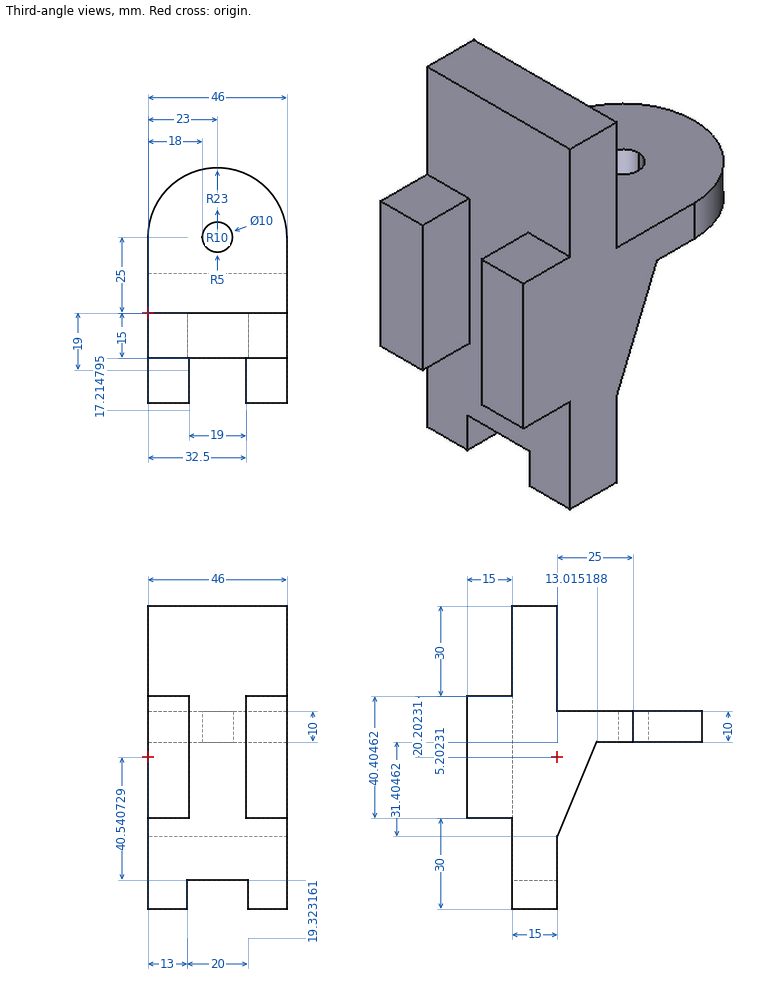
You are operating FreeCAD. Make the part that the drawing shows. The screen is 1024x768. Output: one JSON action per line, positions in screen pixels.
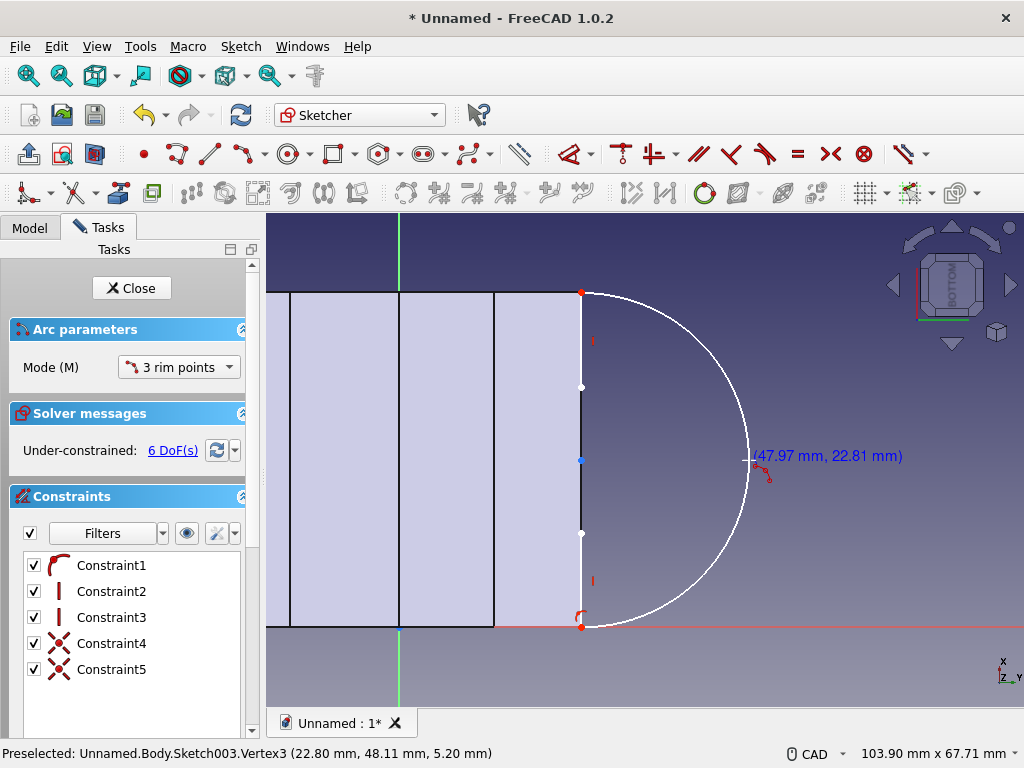
{"action": "left_click", "coordinate": [581, 388]}
{"action": "left_click", "coordinate": [581, 534]}
{"action": "left_click", "coordinate": [654, 460]}
{"action": "key", "text": "Escape"}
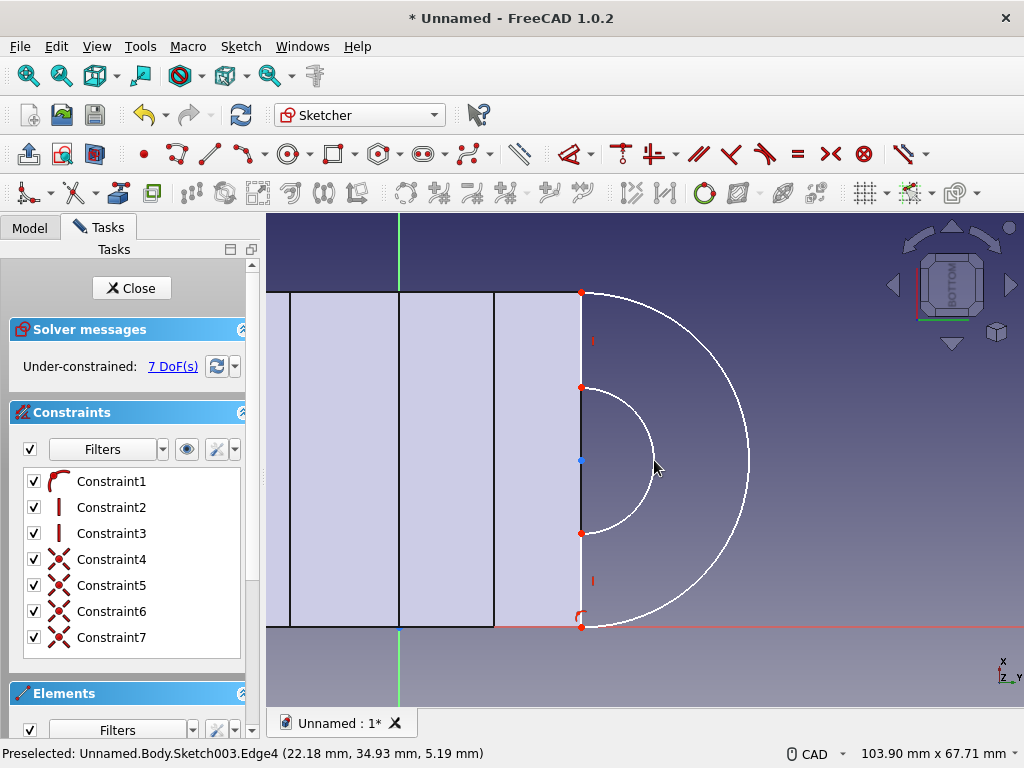
{"action": "left_click", "coordinate": [717, 559]}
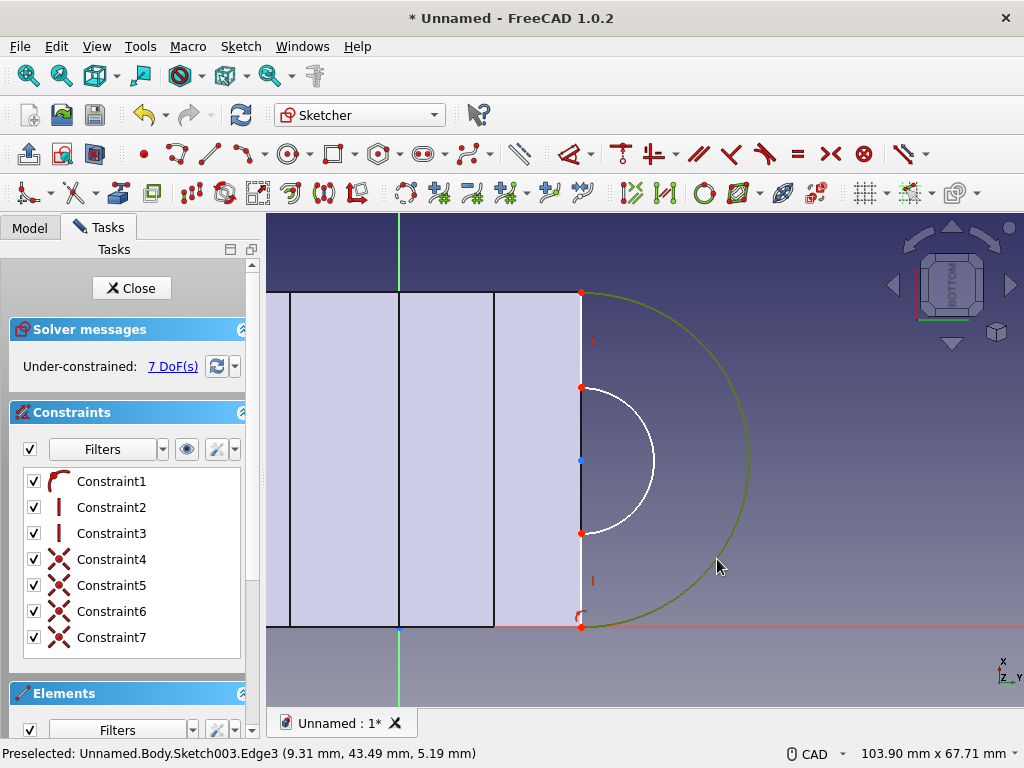
{"action": "left_click", "coordinate": [640, 504]}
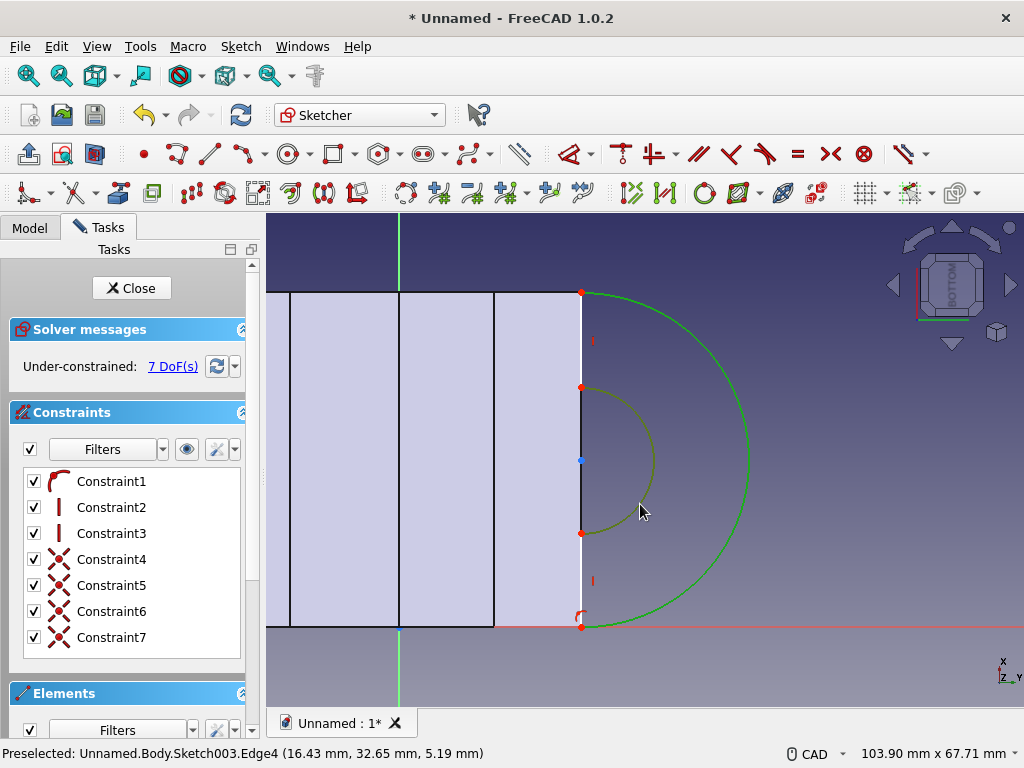
{"action": "key", "text": "c"}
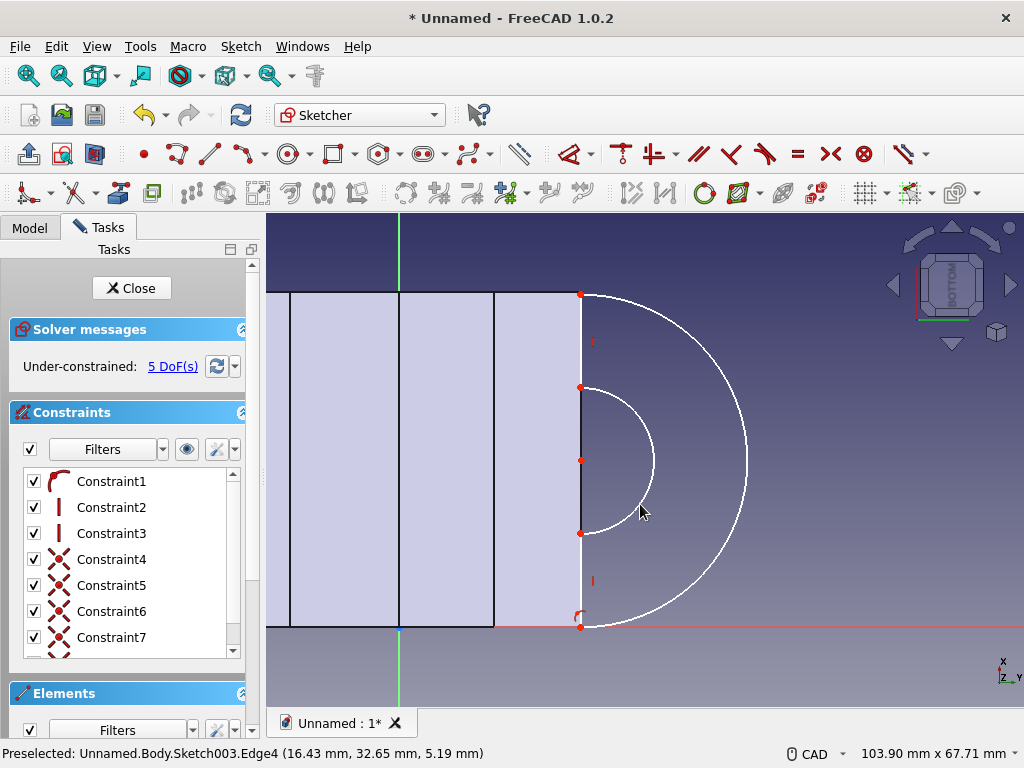
{"action": "left_click", "coordinate": [568, 154]}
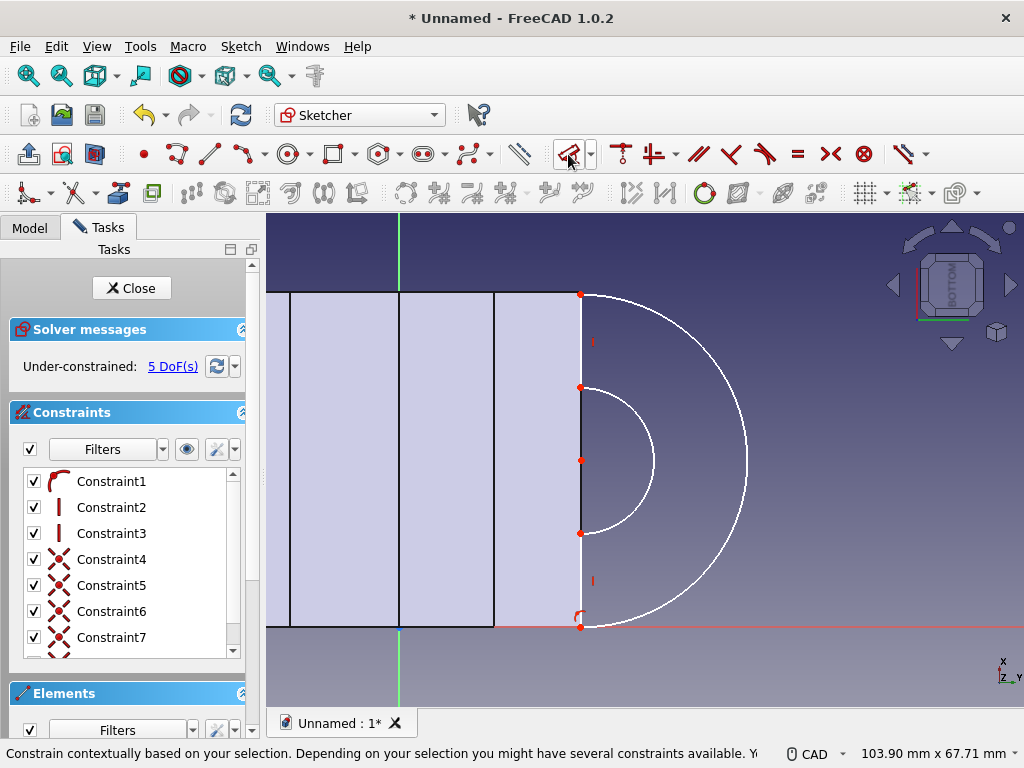
{"action": "left_click", "coordinate": [716, 559]}
{"action": "left_click", "coordinate": [742, 578]}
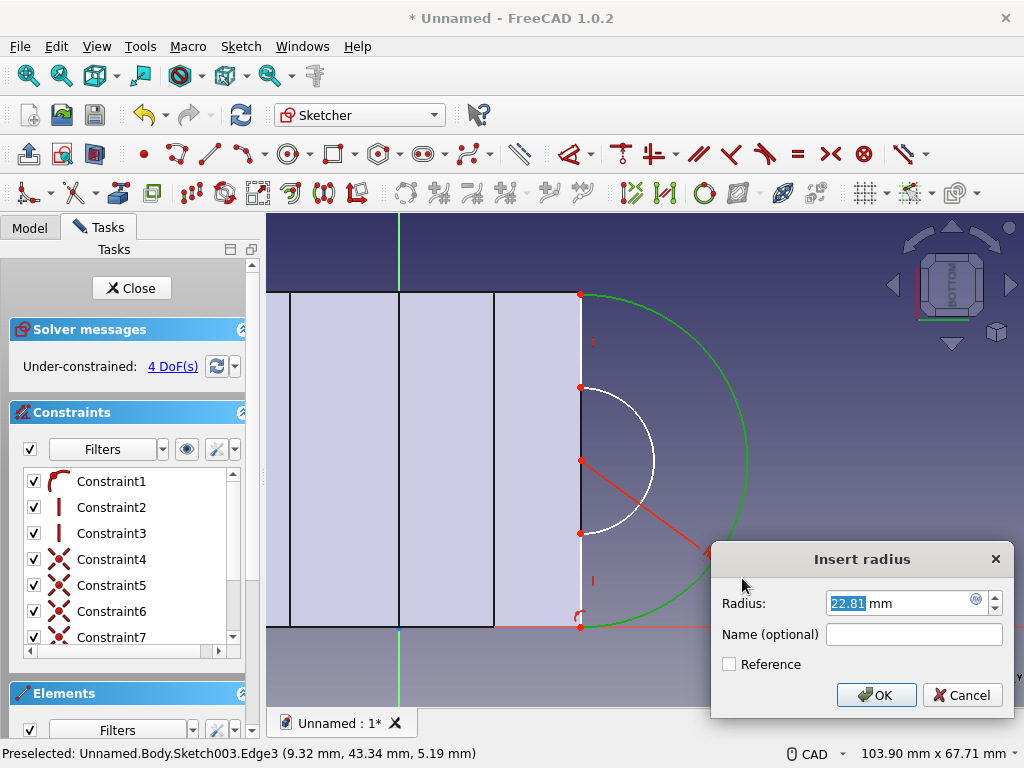
{"action": "type", "text": "23"}
{"action": "key", "text": "Return"}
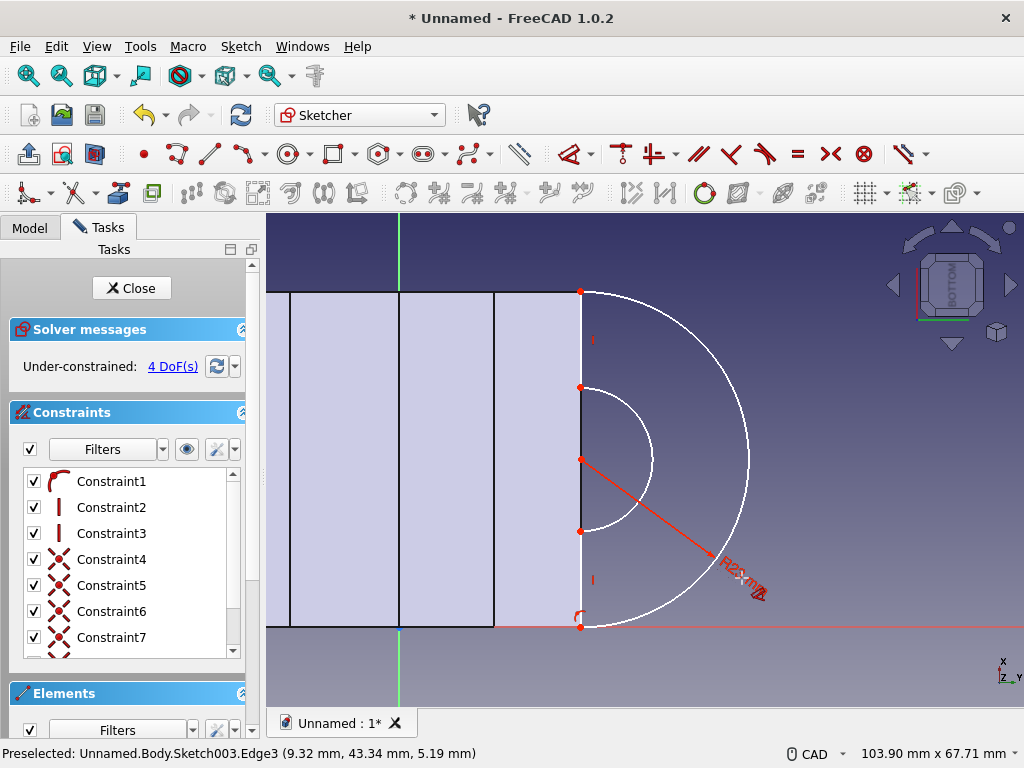
{"action": "left_click", "coordinate": [639, 502]}
{"action": "left_click", "coordinate": [665, 521]}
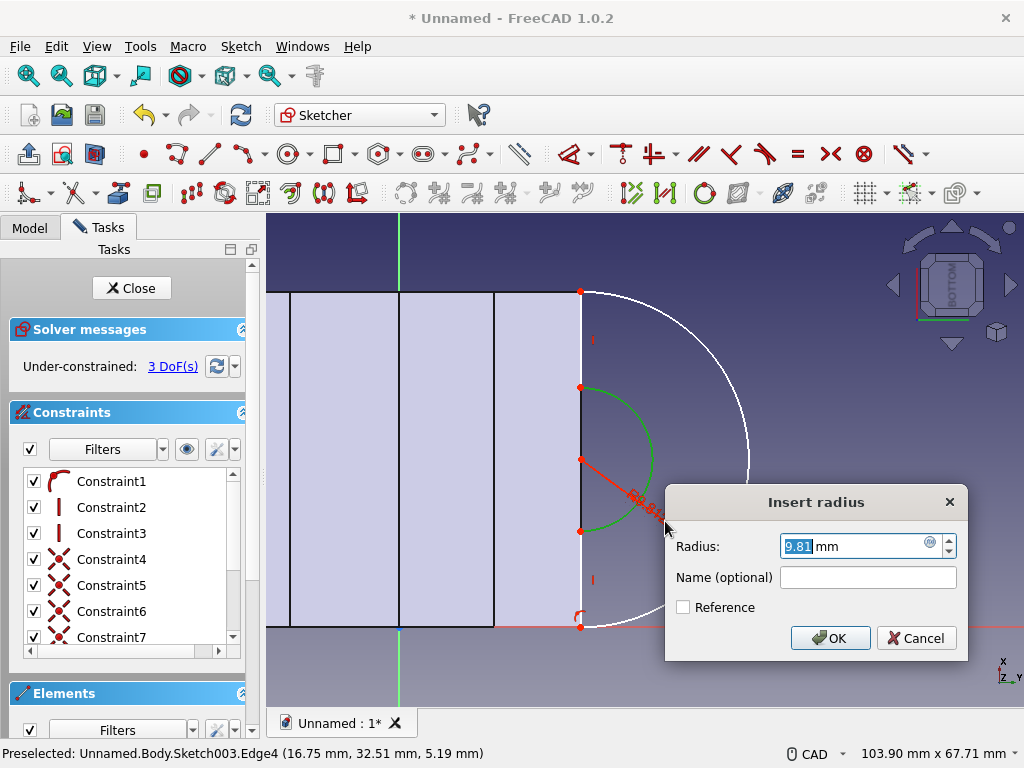
{"action": "type", "text": "10"}
{"action": "key", "text": "Return"}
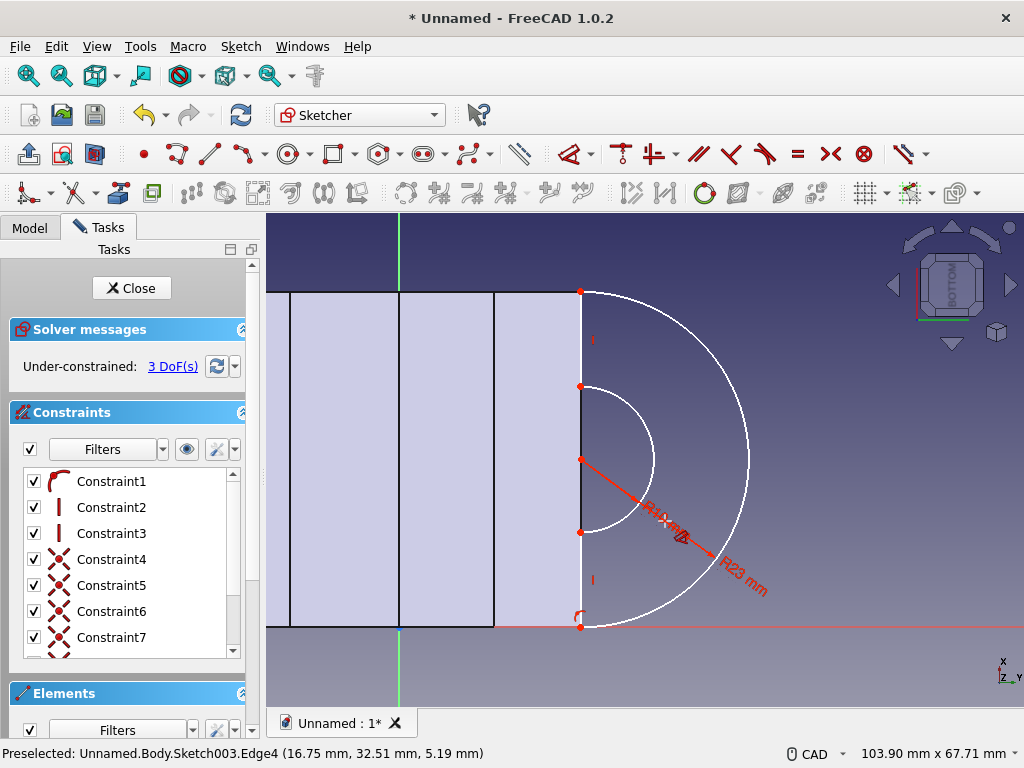
{"action": "left_click", "coordinate": [581, 533]}
{"action": "left_click", "coordinate": [490, 661]}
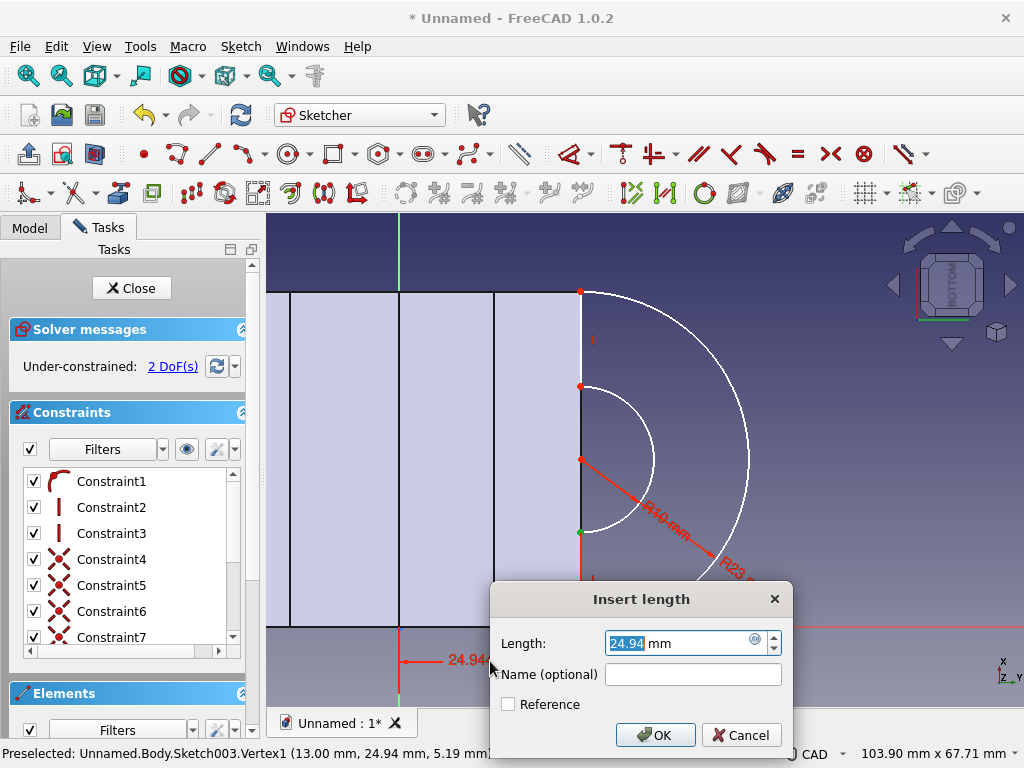
{"action": "type", "text": "25"}
{"action": "key", "text": "Return"}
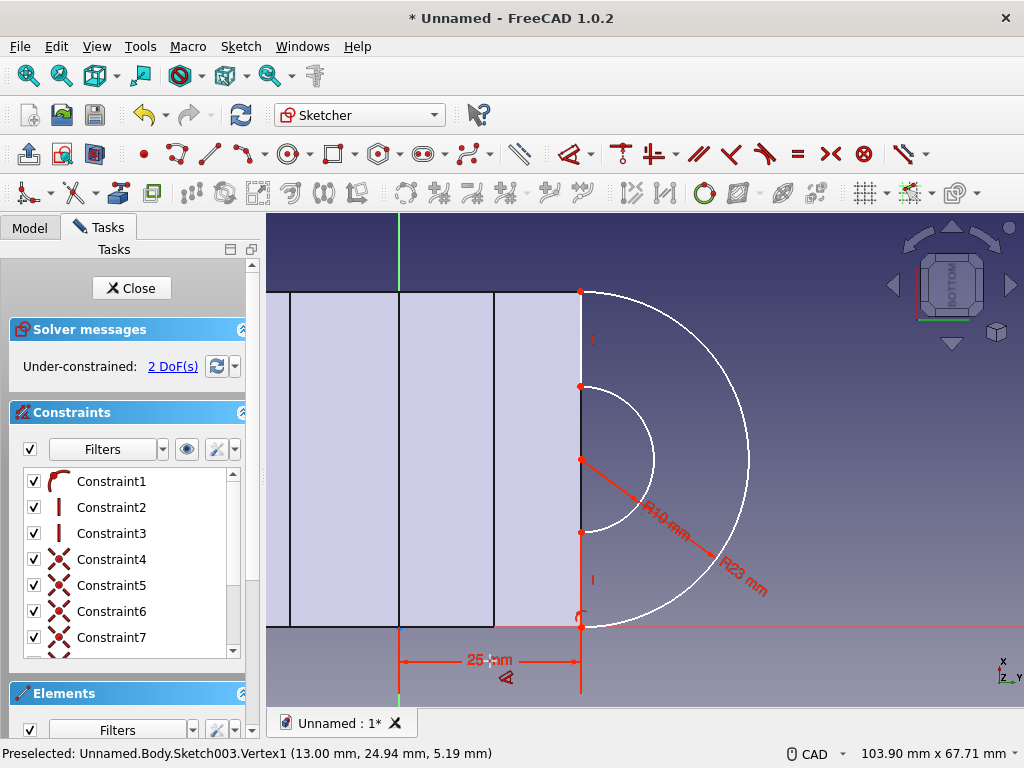
{"action": "left_click", "coordinate": [581, 292]}
{"action": "left_click", "coordinate": [490, 258]}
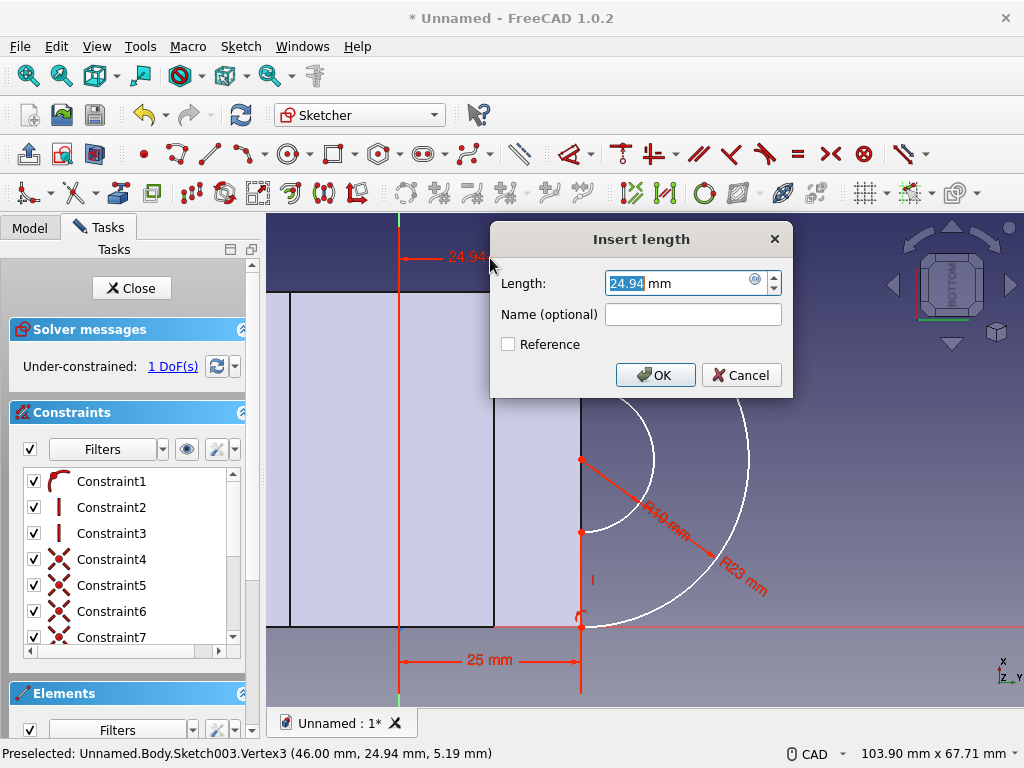
{"action": "type", "text": "25"}
{"action": "key", "text": "Return"}